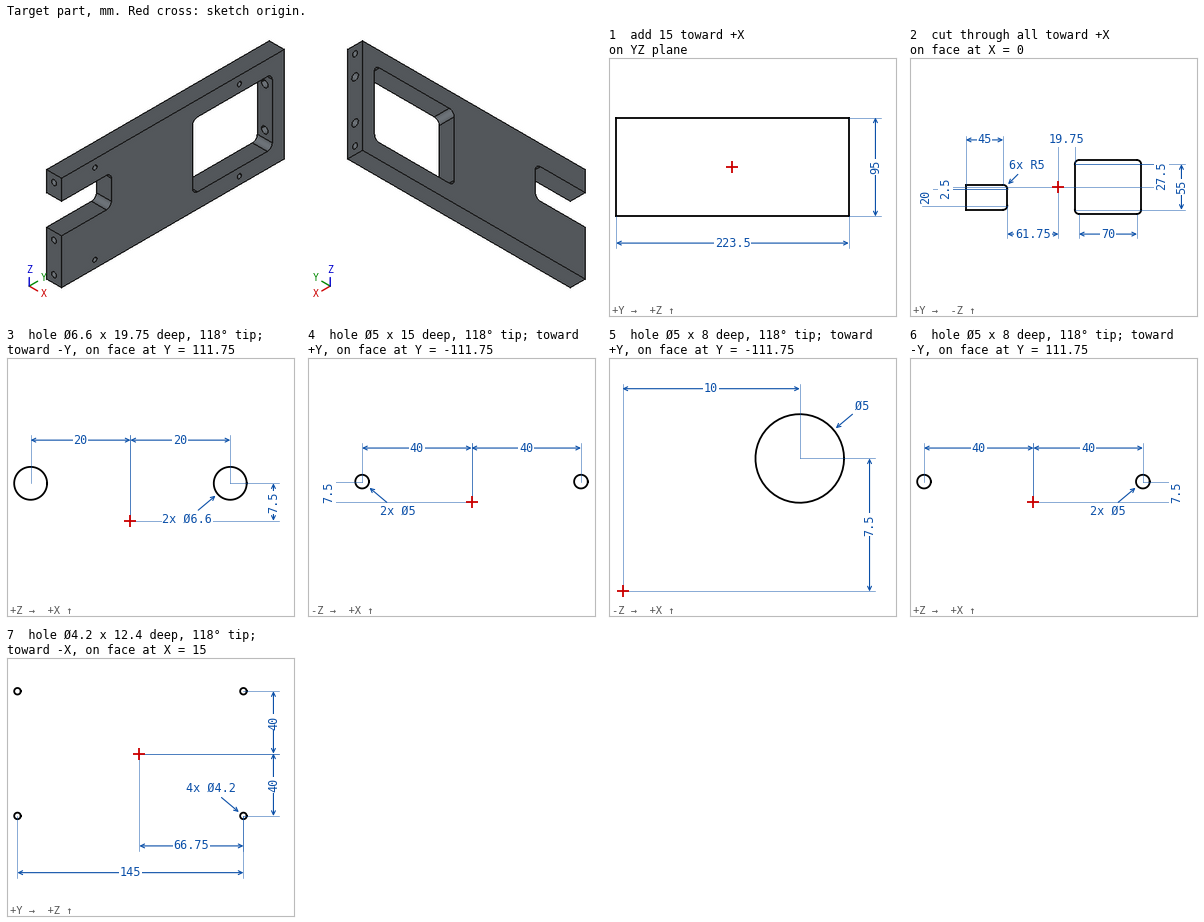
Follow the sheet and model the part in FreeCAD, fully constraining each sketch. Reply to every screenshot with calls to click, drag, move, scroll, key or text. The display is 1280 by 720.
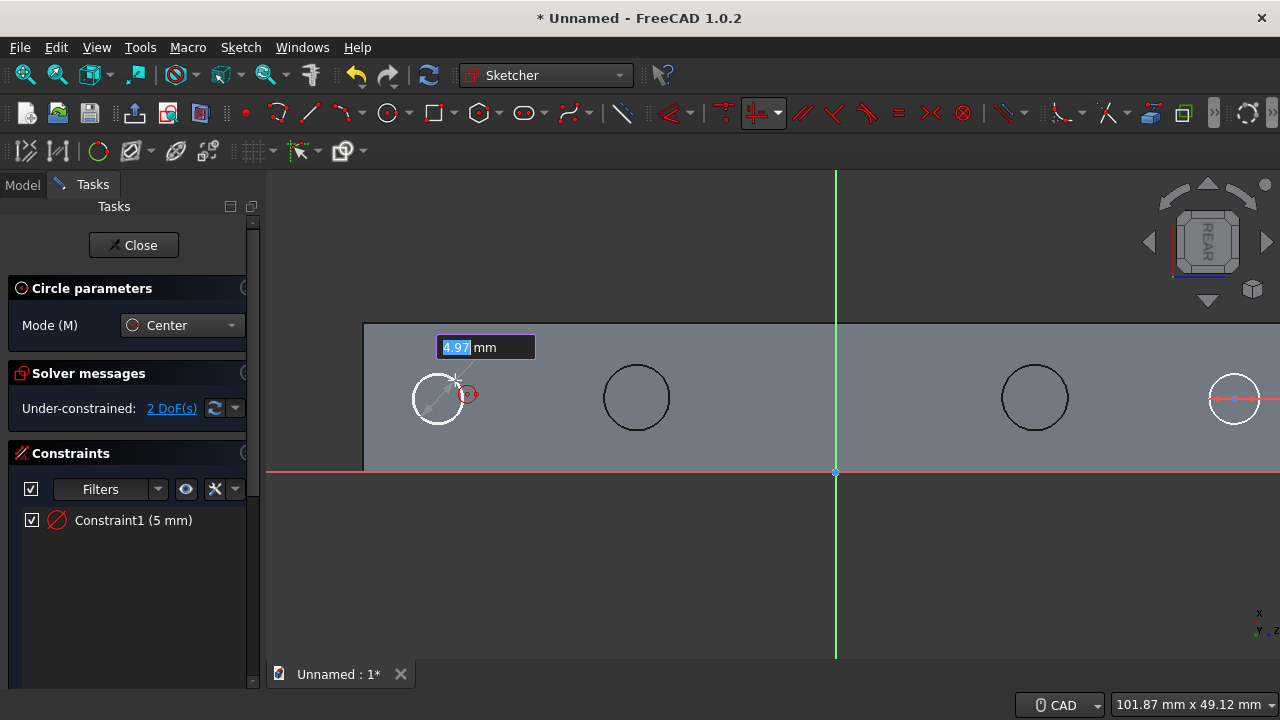
text(5)
key(Return)
key(Escape)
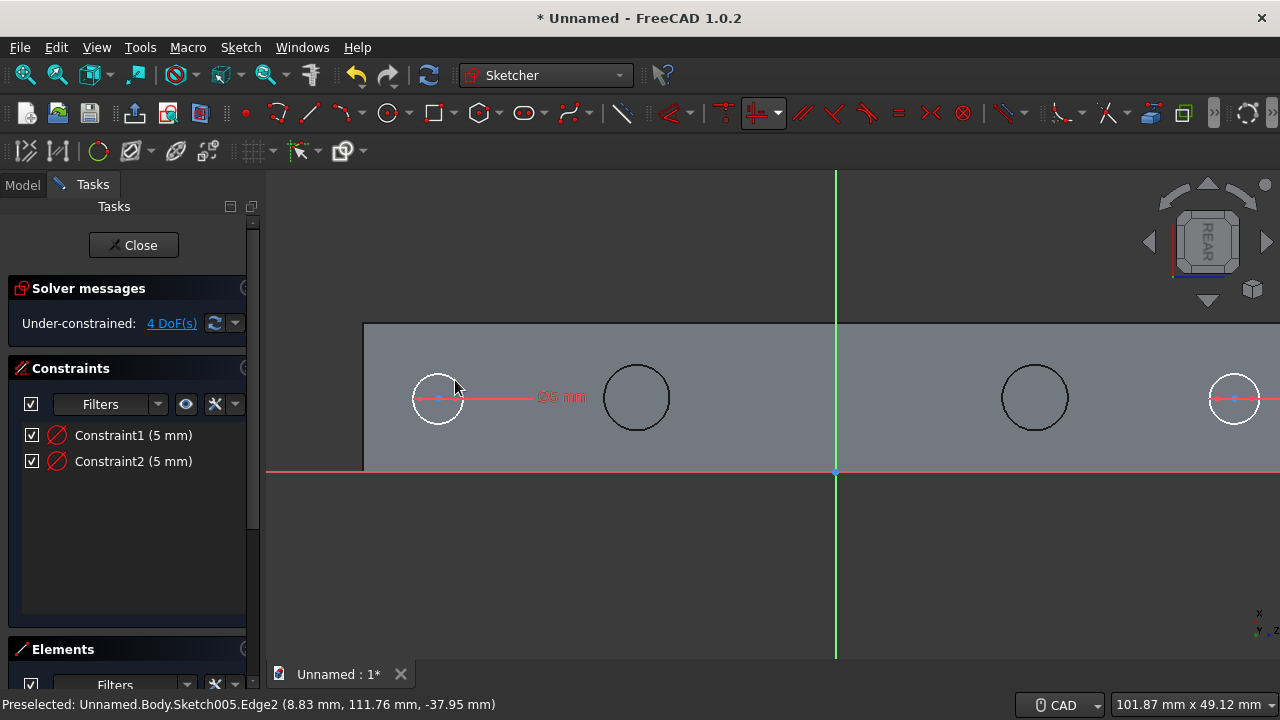
scroll(437, 398, down, 2)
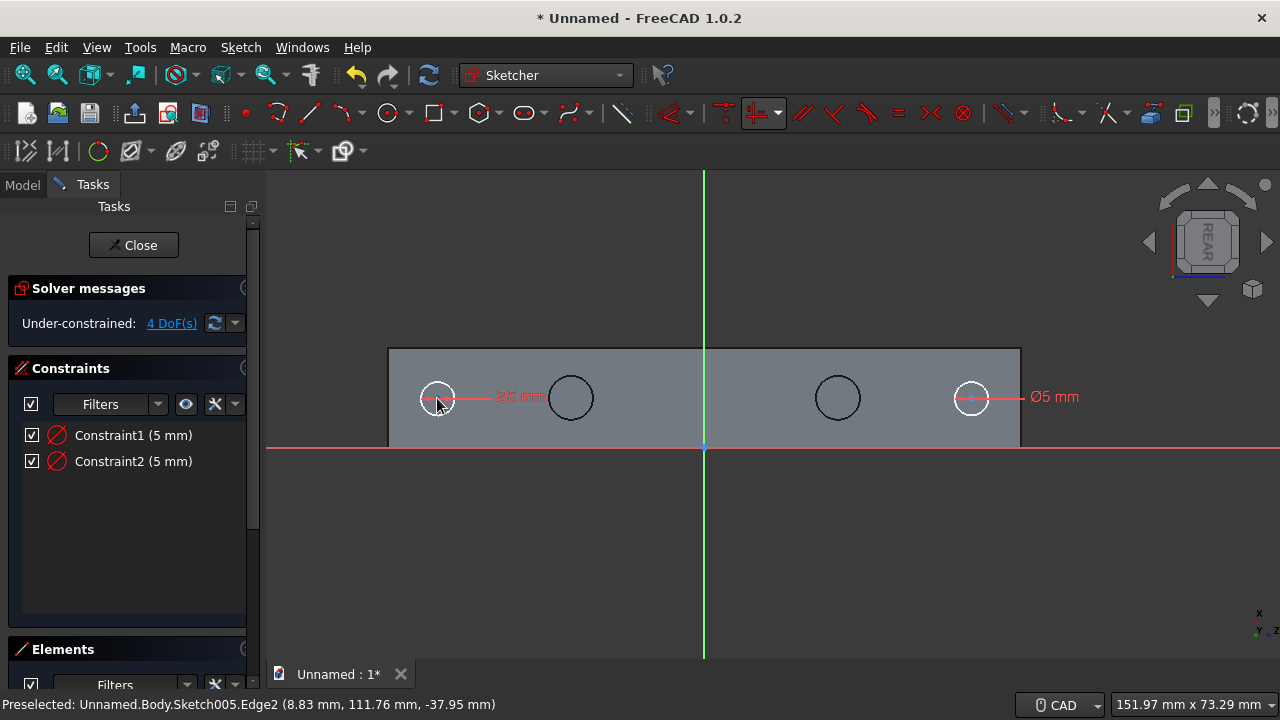
click(972, 399)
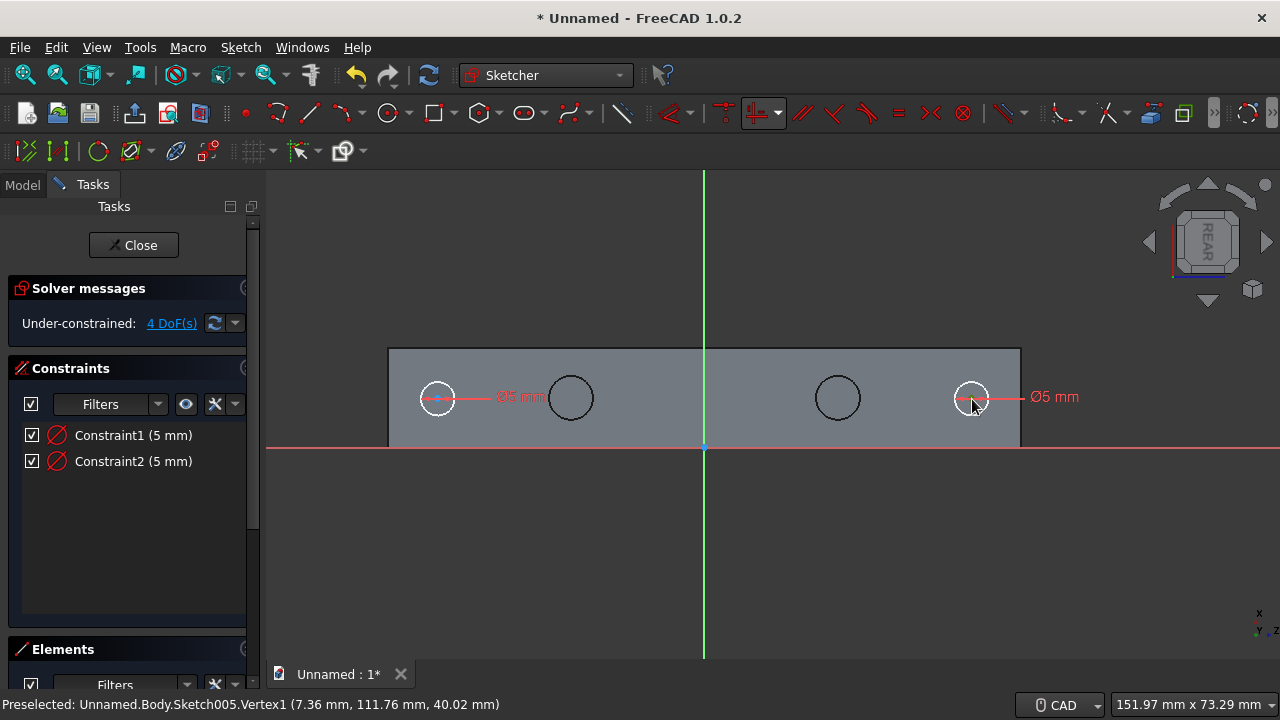
click(438, 399)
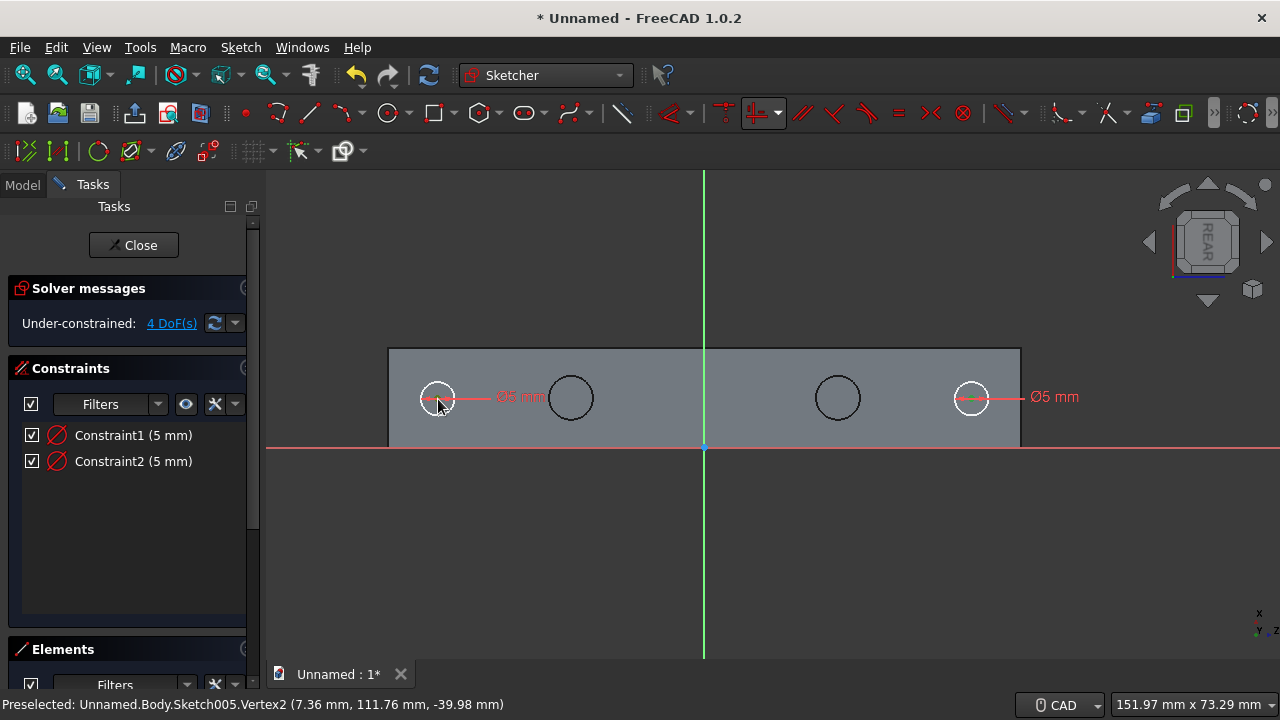
click(780, 114)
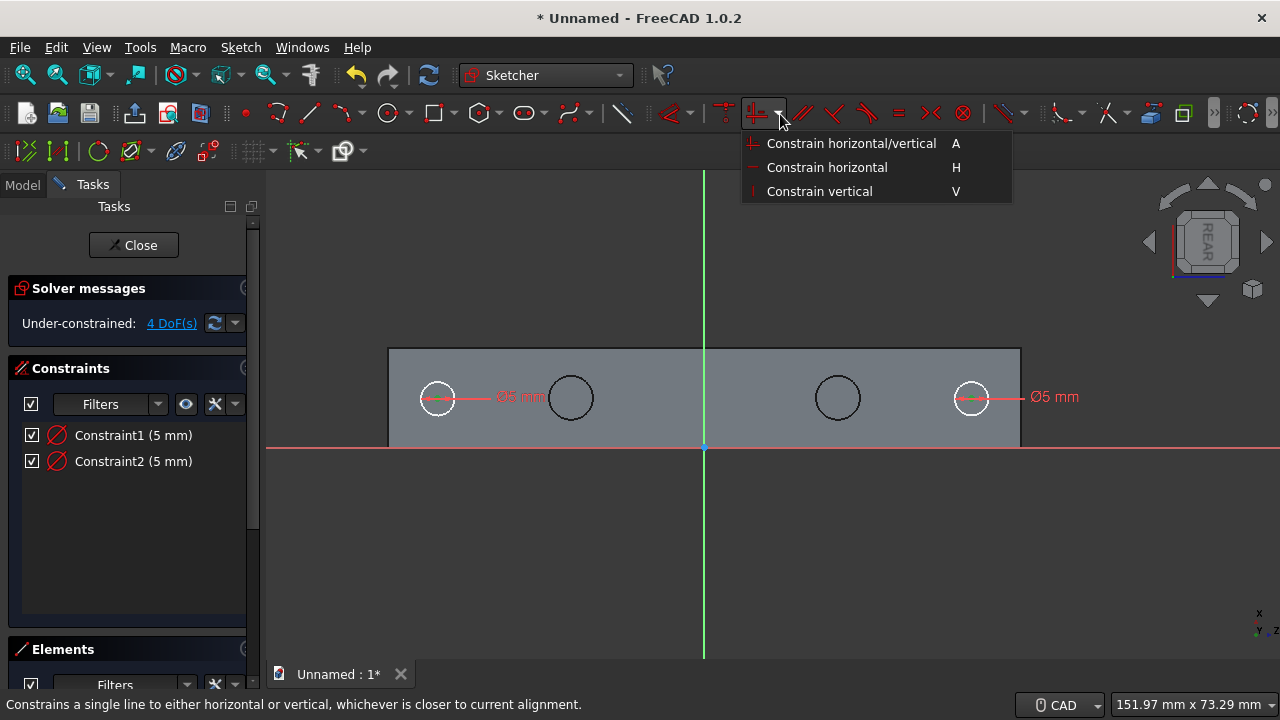
click(877, 167)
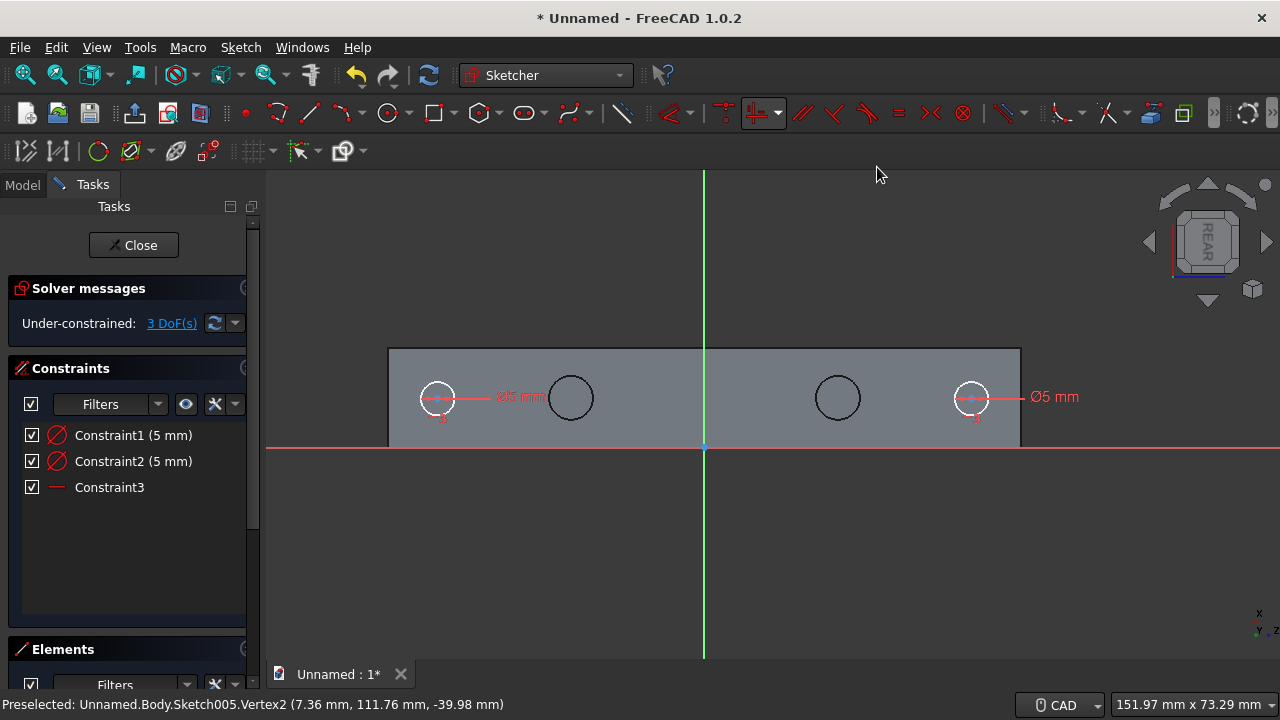
click(670, 114)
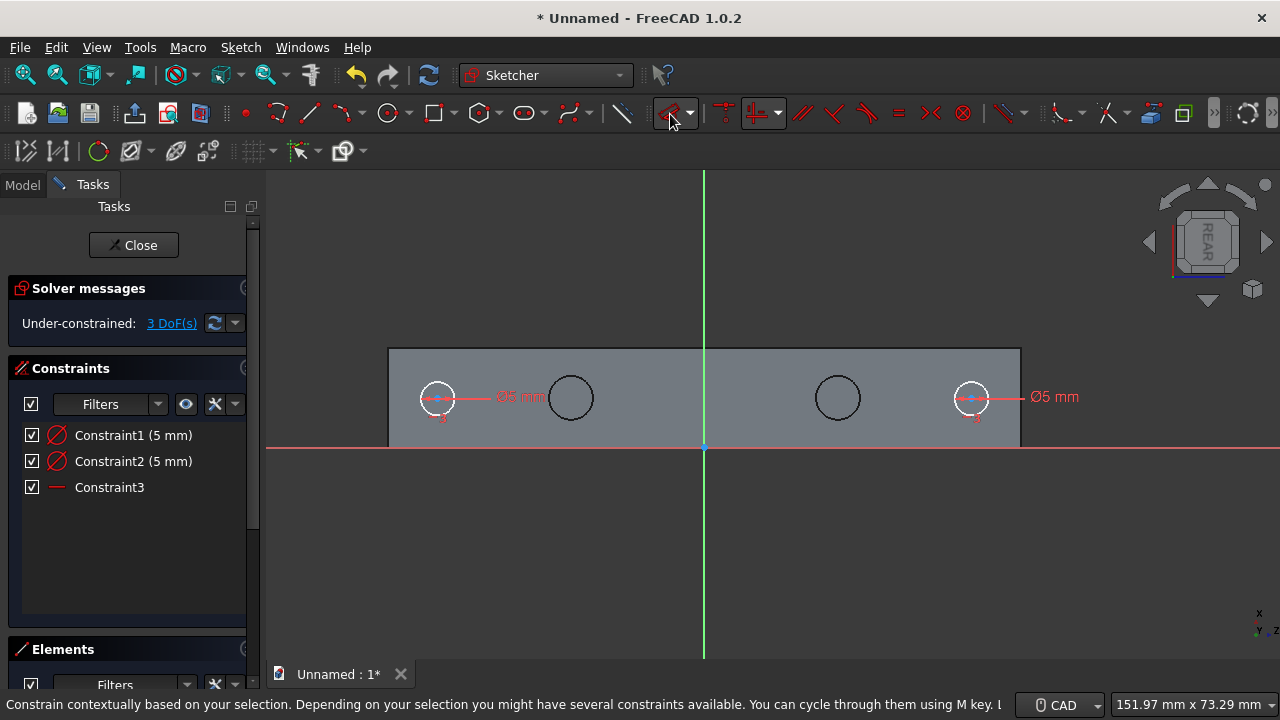
click(972, 399)
click(838, 482)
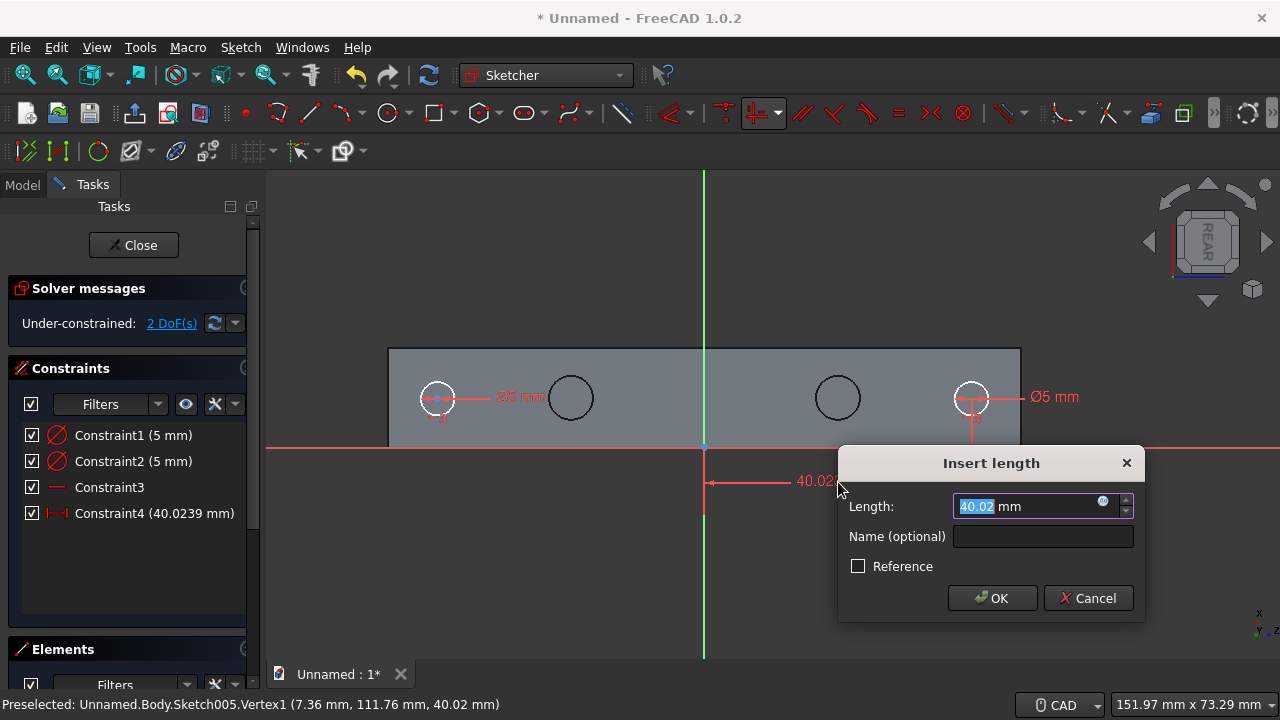
text(40)
key(Return)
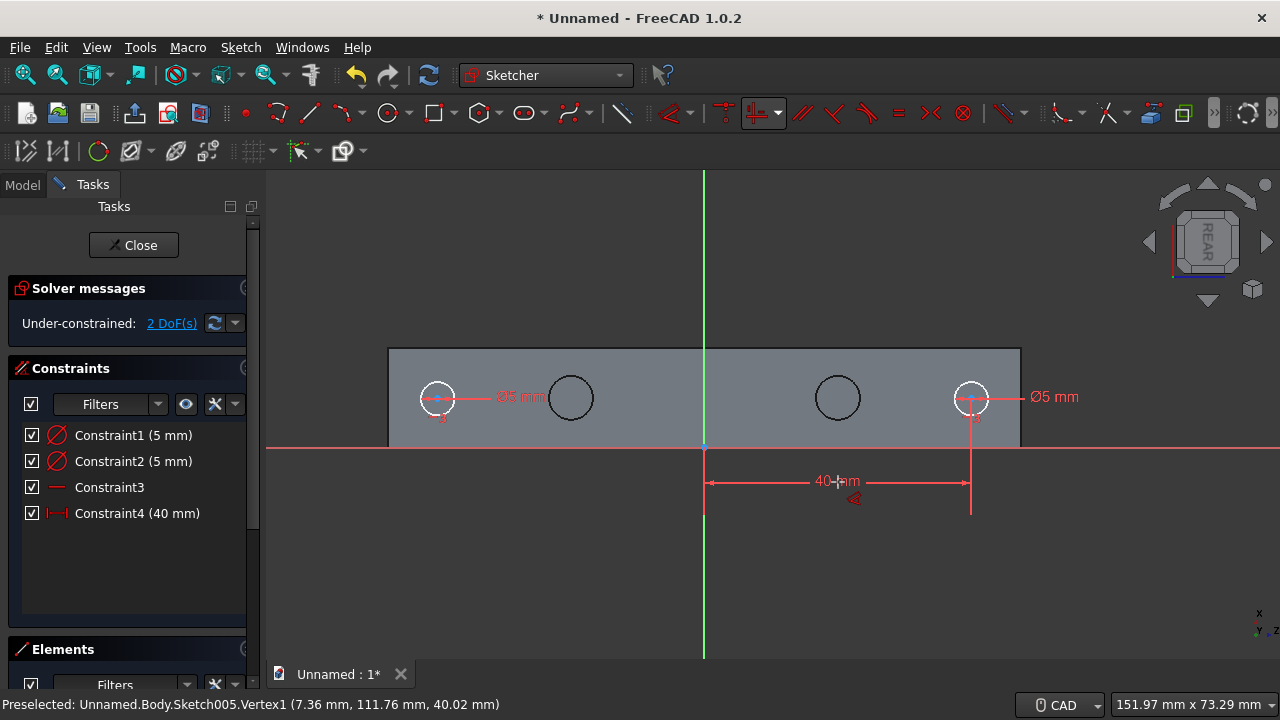
click(438, 399)
click(571, 482)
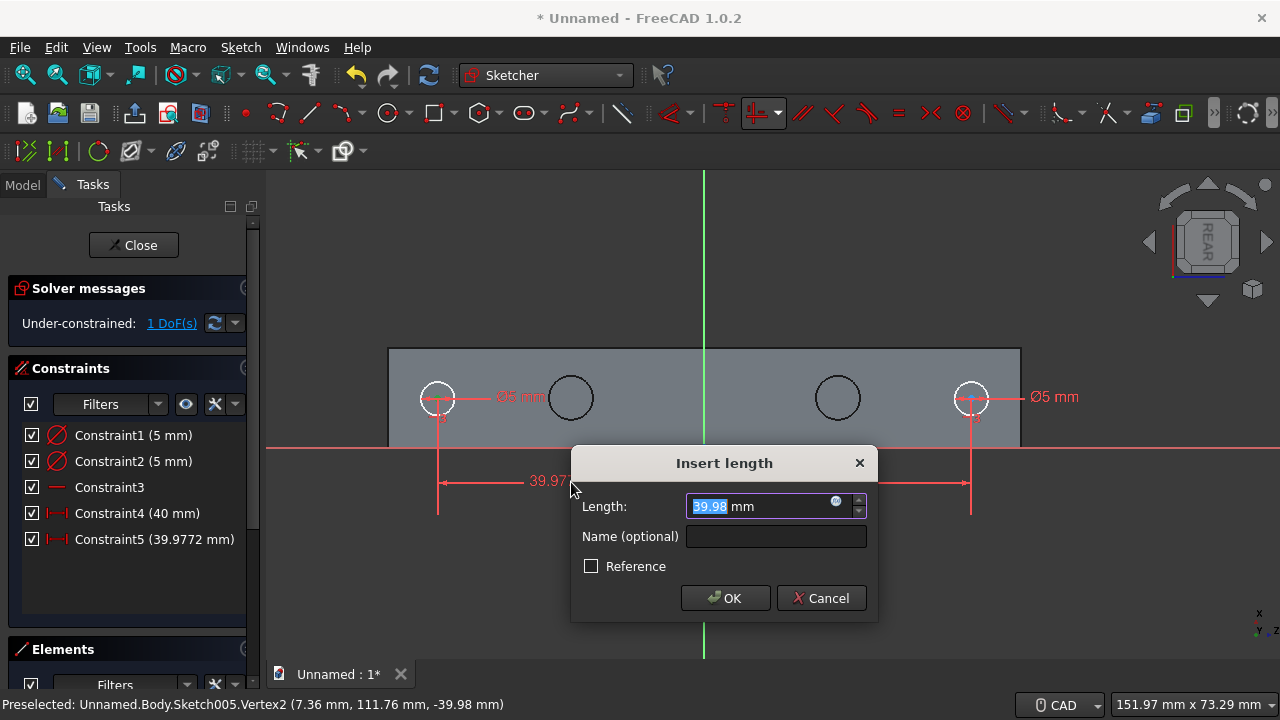
text(40)
key(Return)